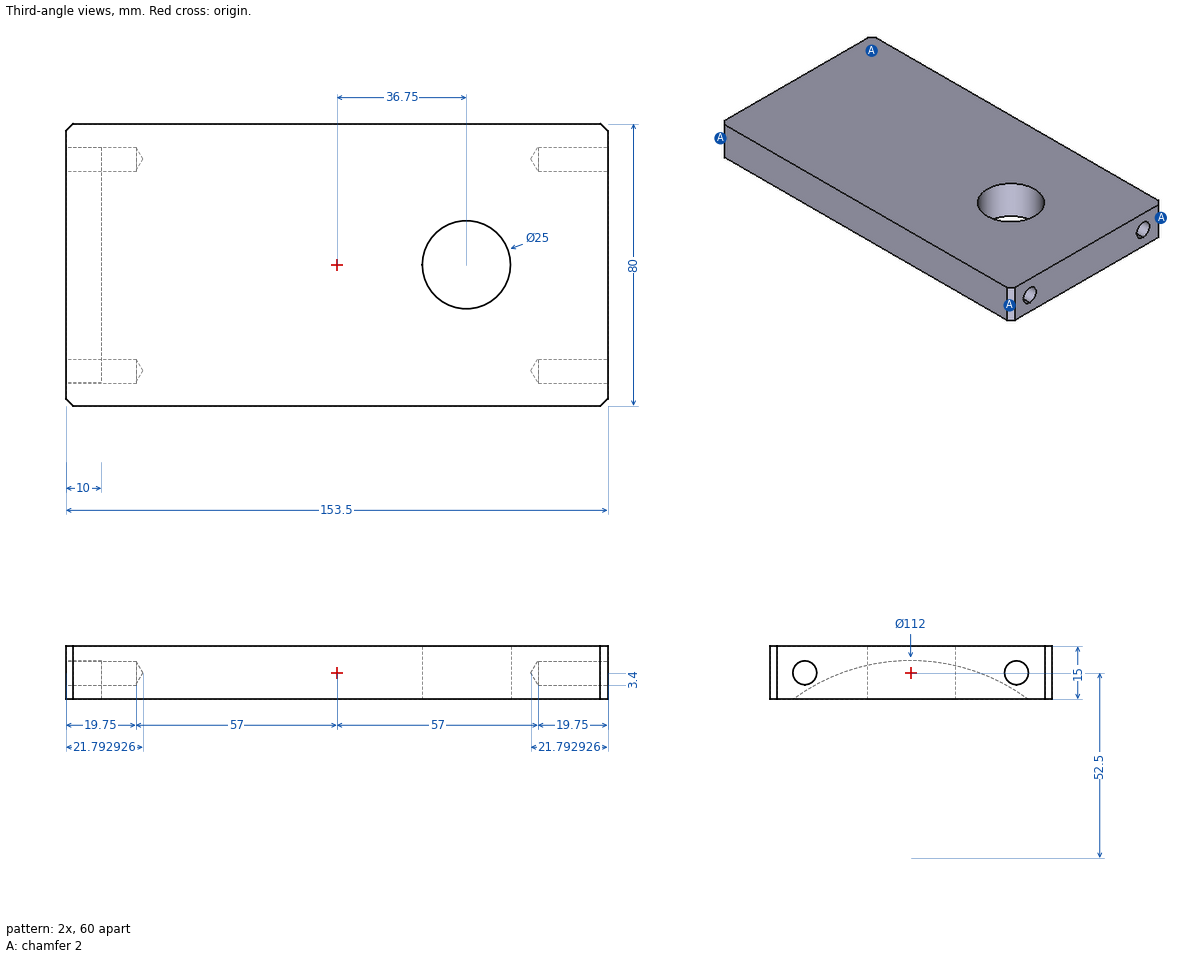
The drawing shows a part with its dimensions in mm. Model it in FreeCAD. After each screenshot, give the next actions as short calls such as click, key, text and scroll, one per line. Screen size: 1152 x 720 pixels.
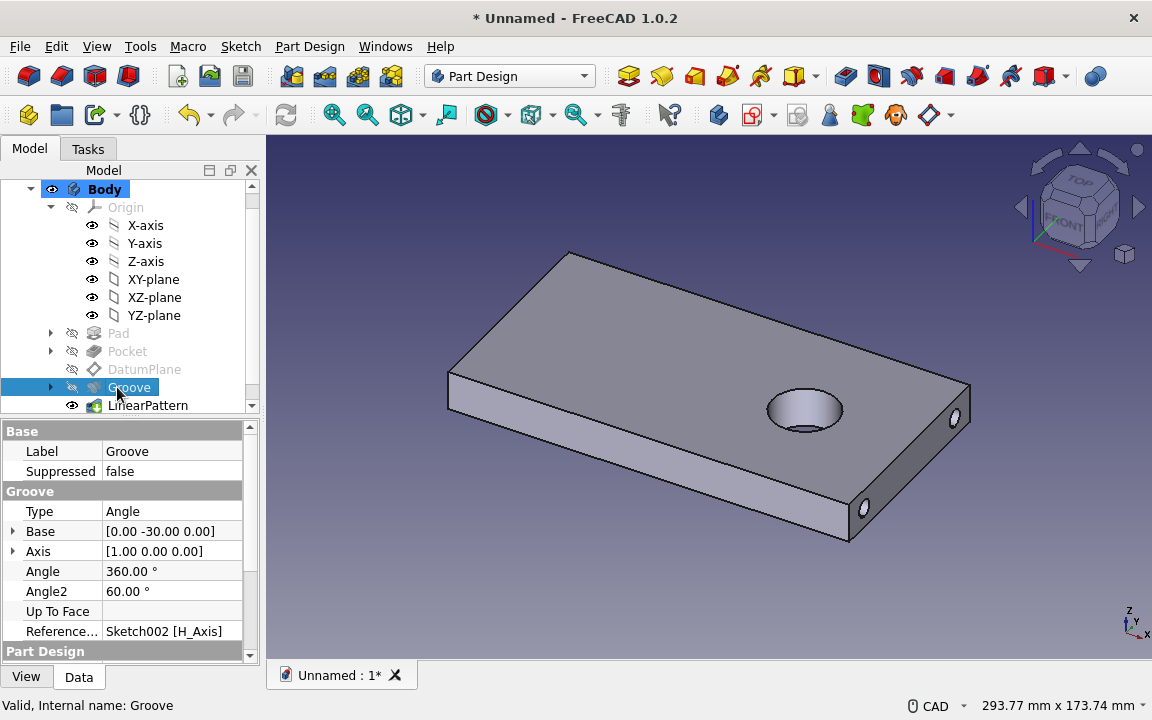
click(292, 76)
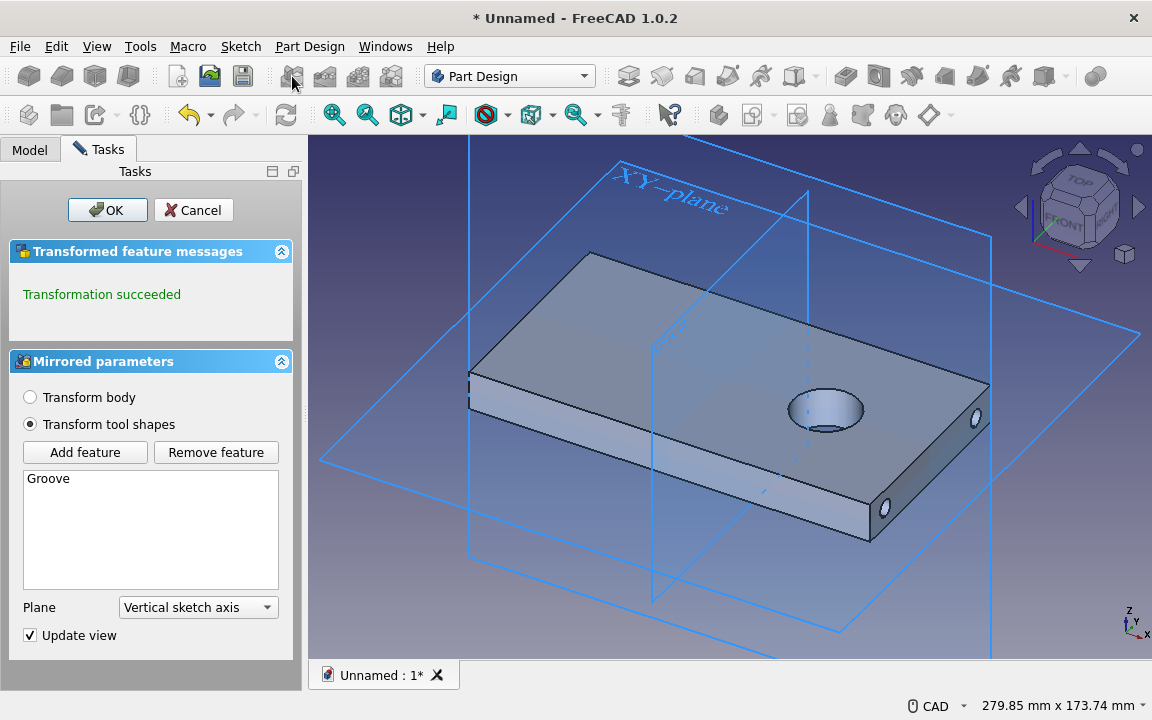
click(199, 608)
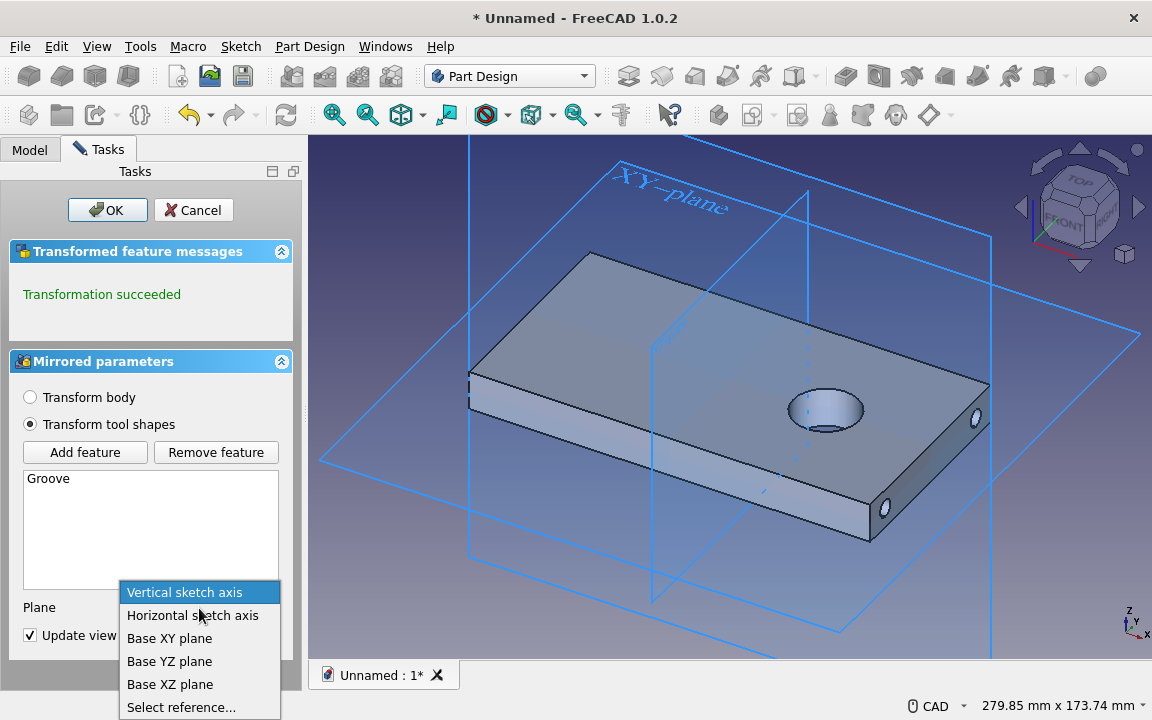
click(198, 662)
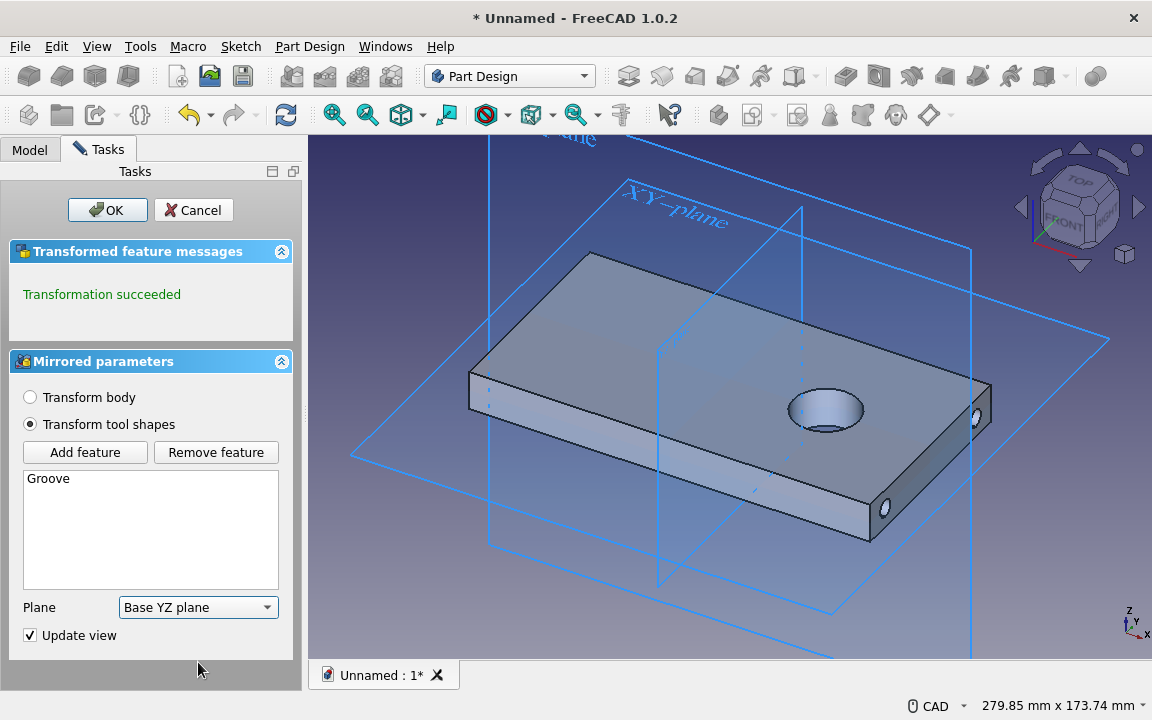
click(108, 210)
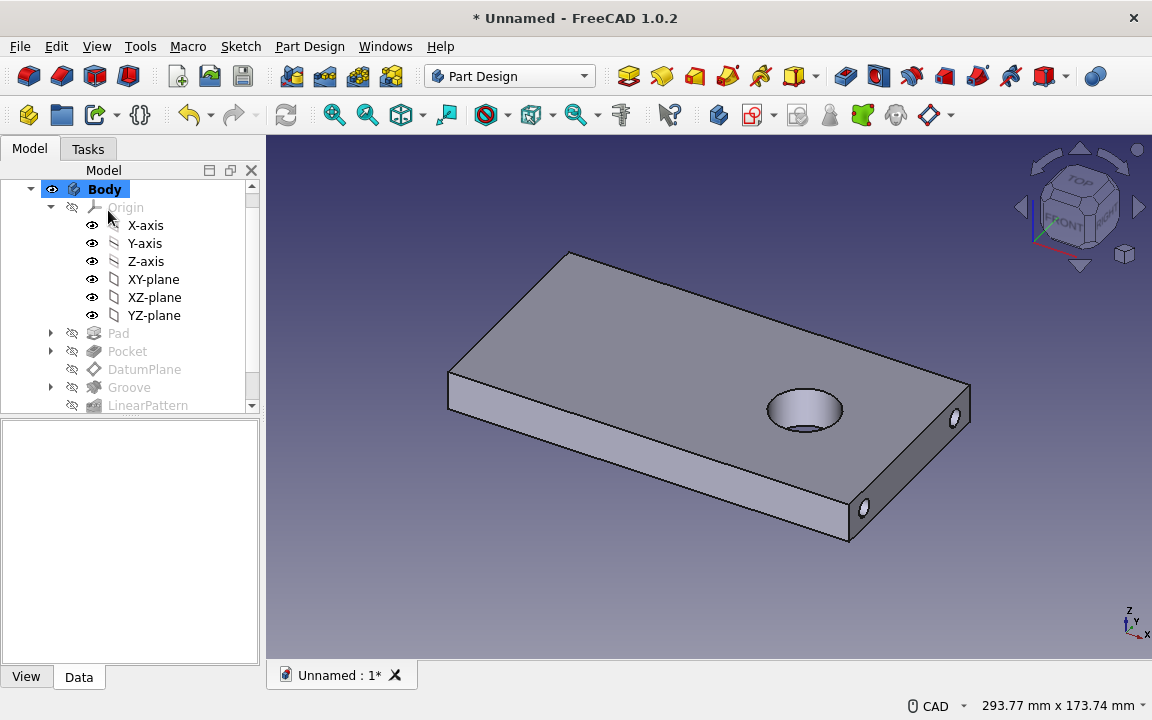
click(137, 297)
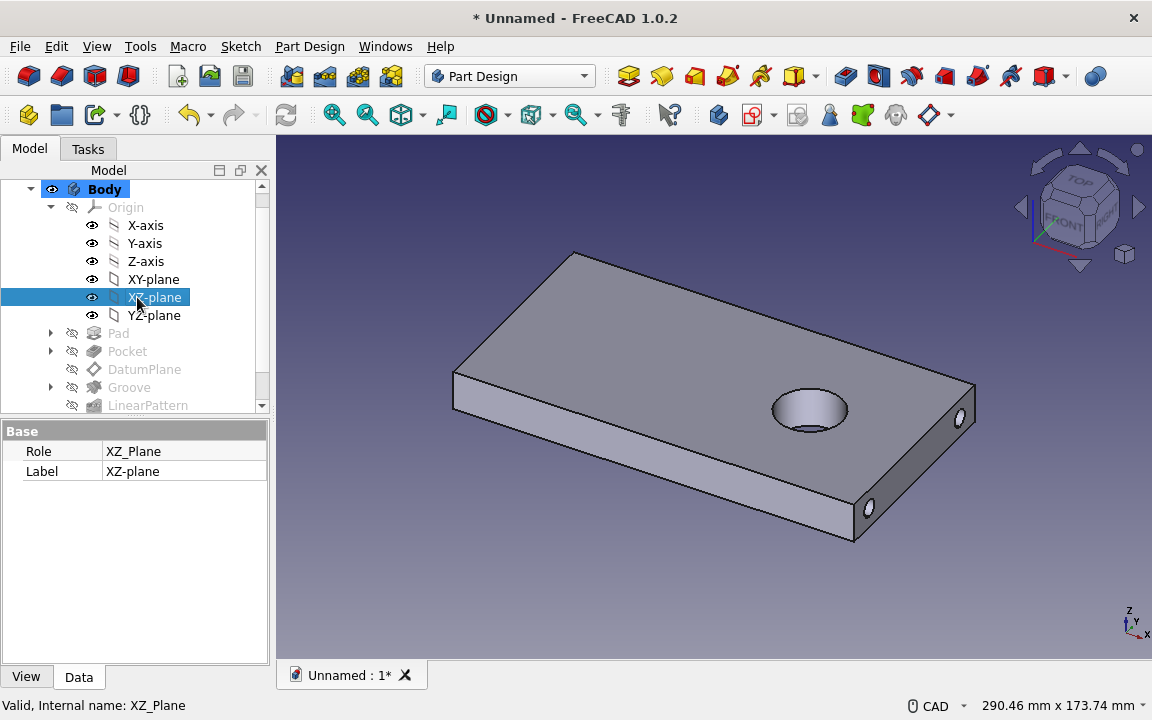
click(928, 116)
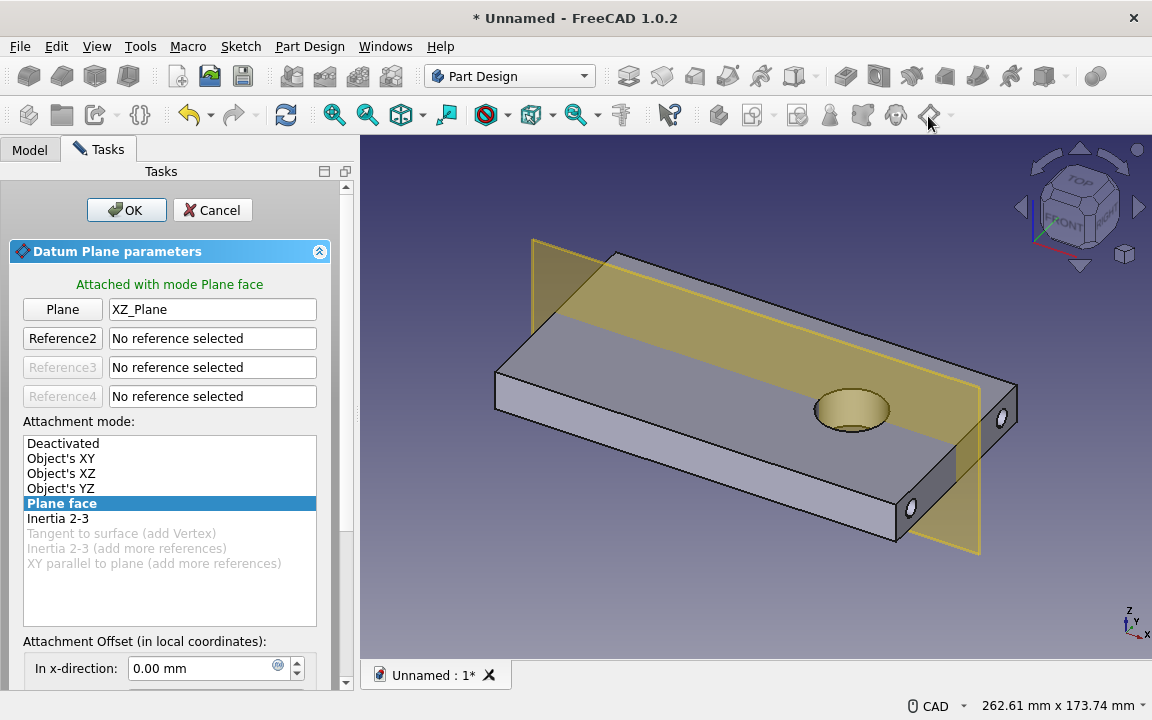
scroll(346, 436, down, 2)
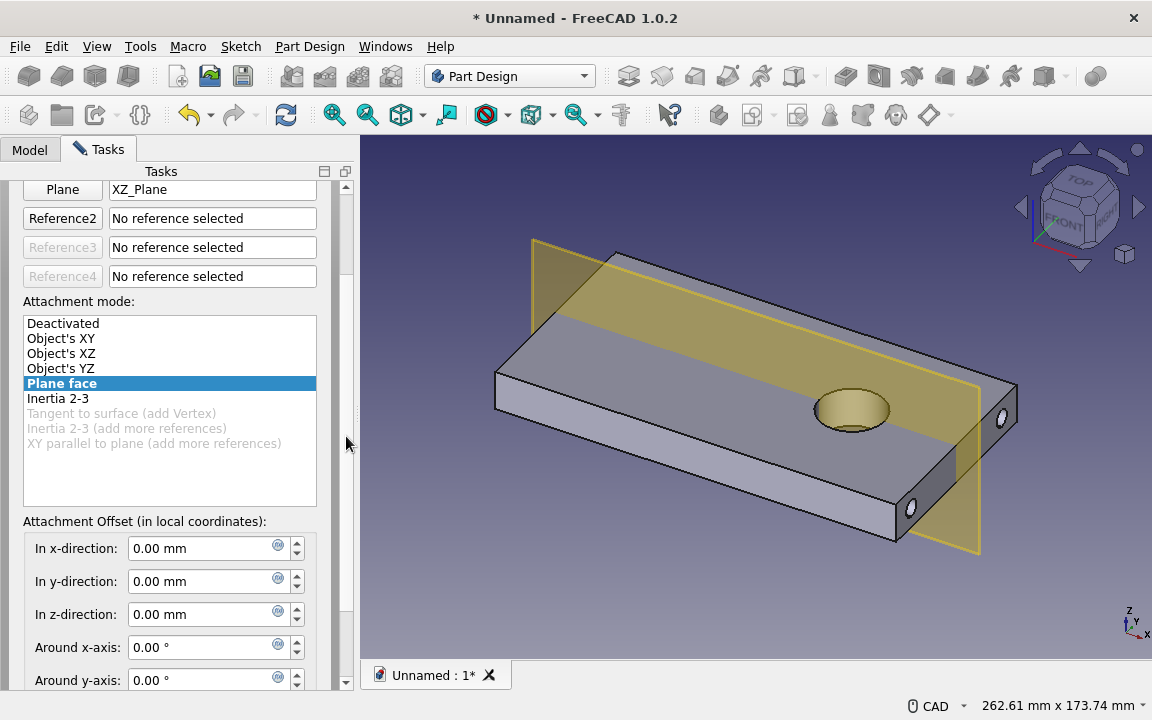
triple_click(210, 614)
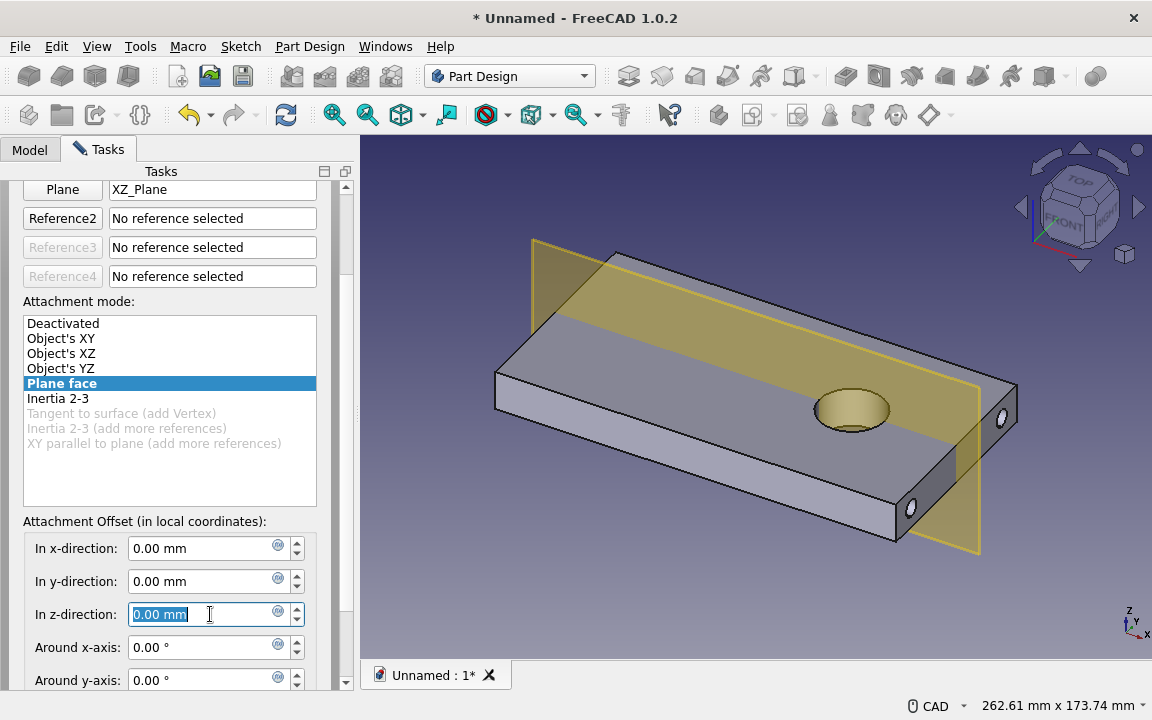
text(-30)
key(Tab)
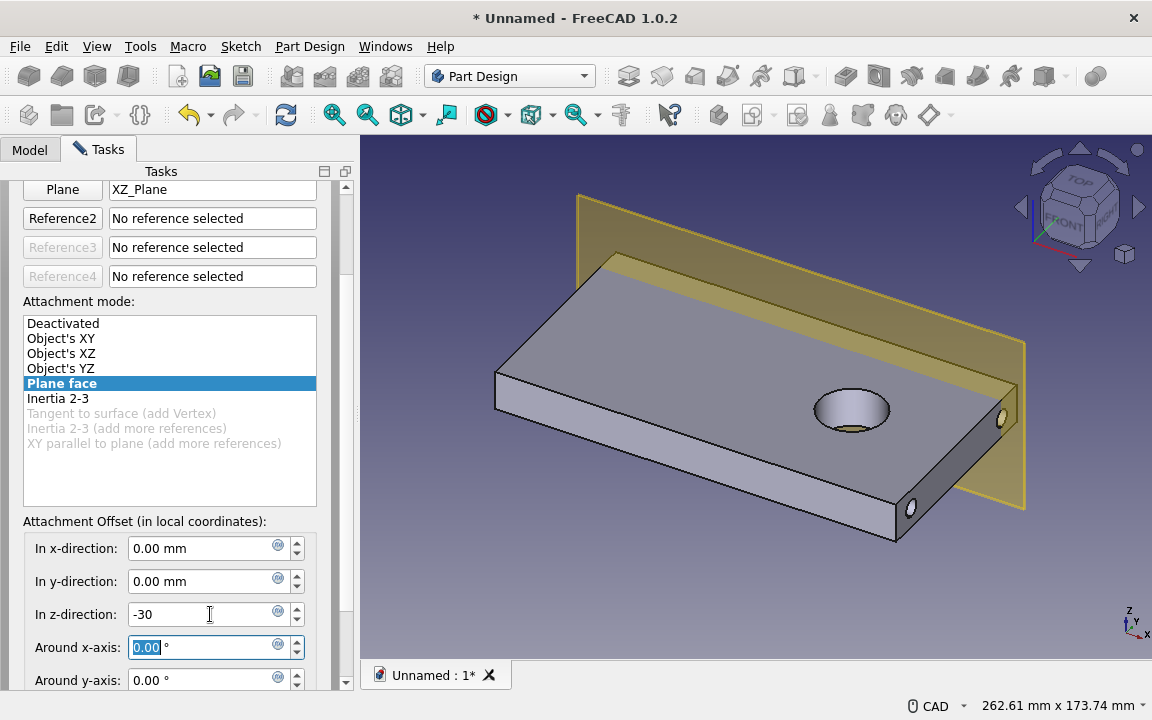
scroll(346, 436, up, 3)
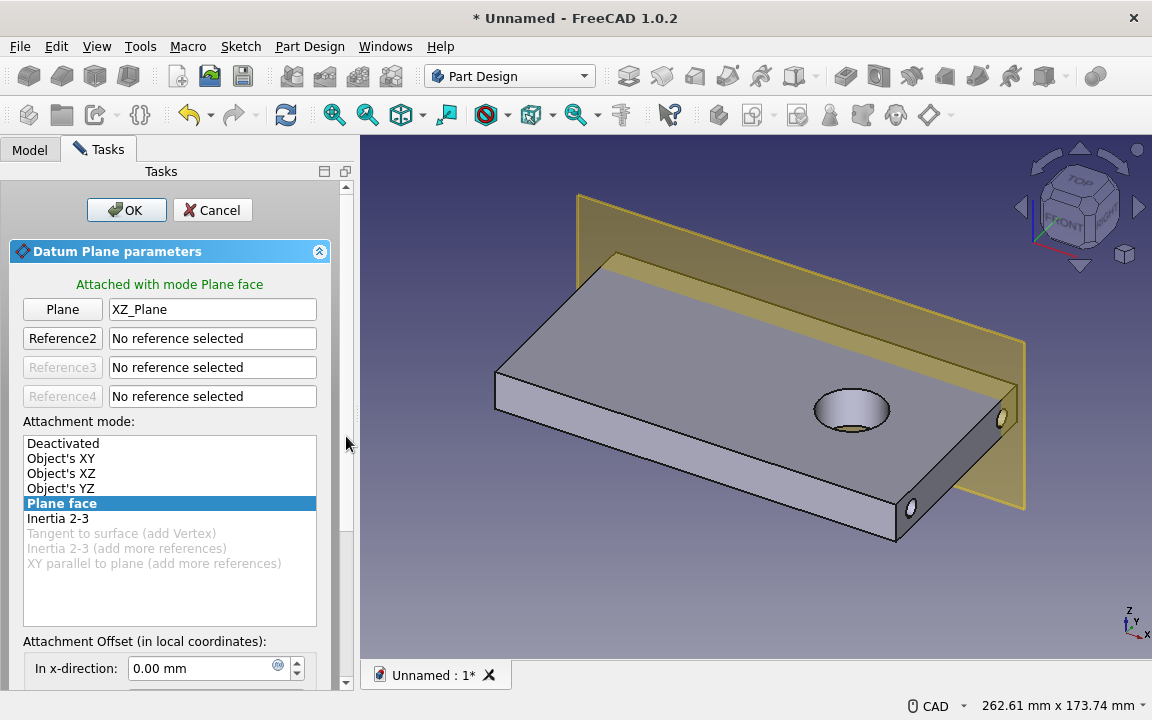
click(127, 210)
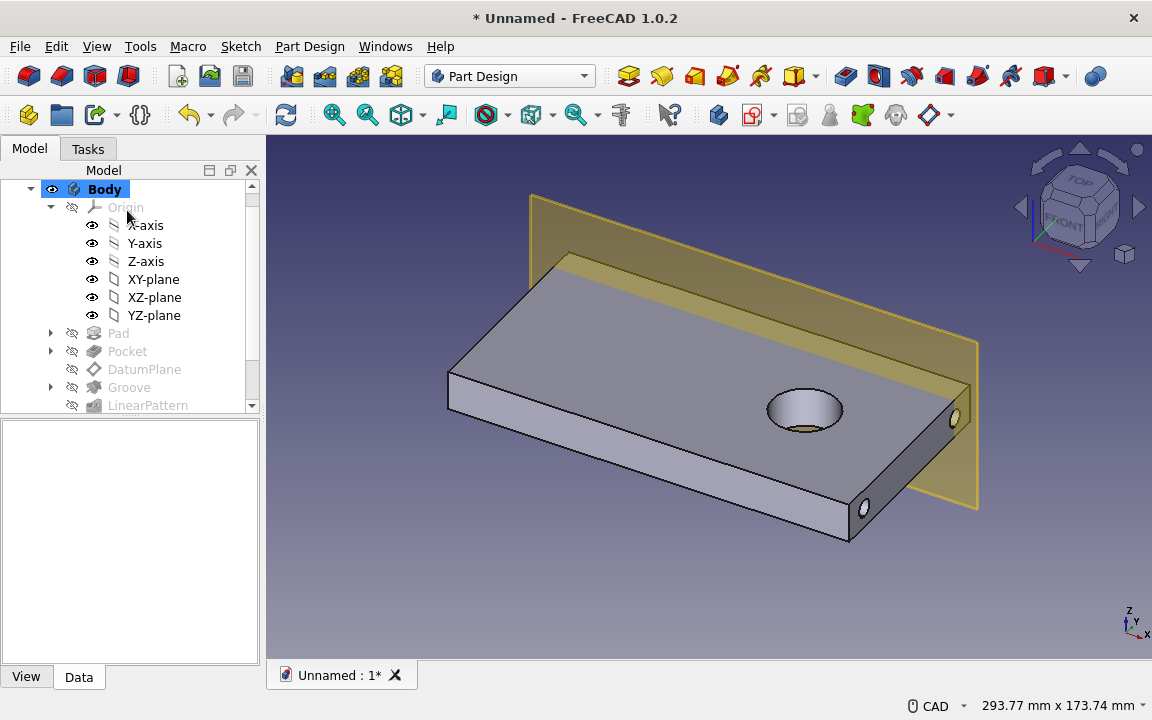
scroll(121, 293, down, 3)